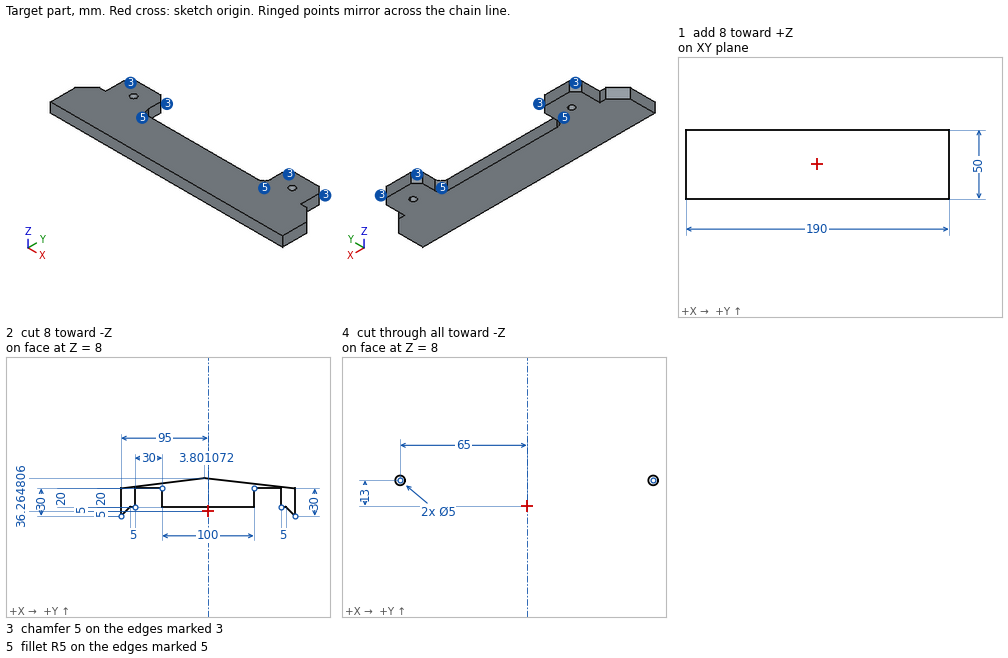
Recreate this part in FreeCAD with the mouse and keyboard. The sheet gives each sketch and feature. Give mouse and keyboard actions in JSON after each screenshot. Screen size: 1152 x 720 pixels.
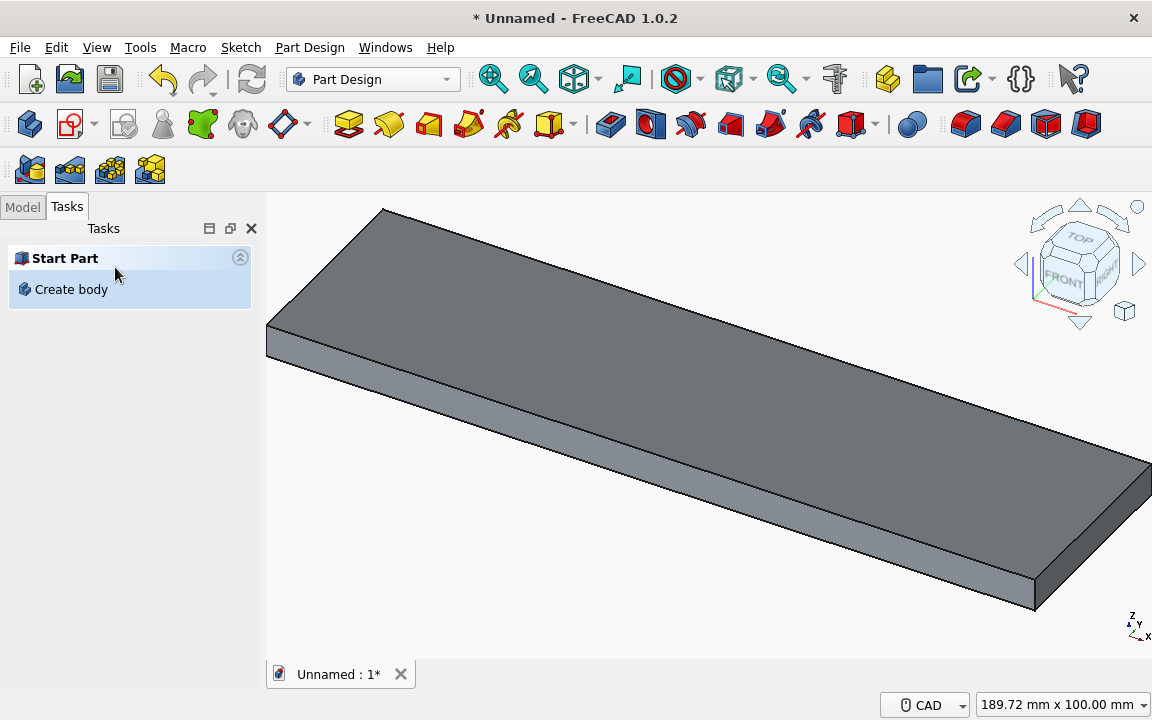
{"action": "left_click", "coordinate": [929, 466]}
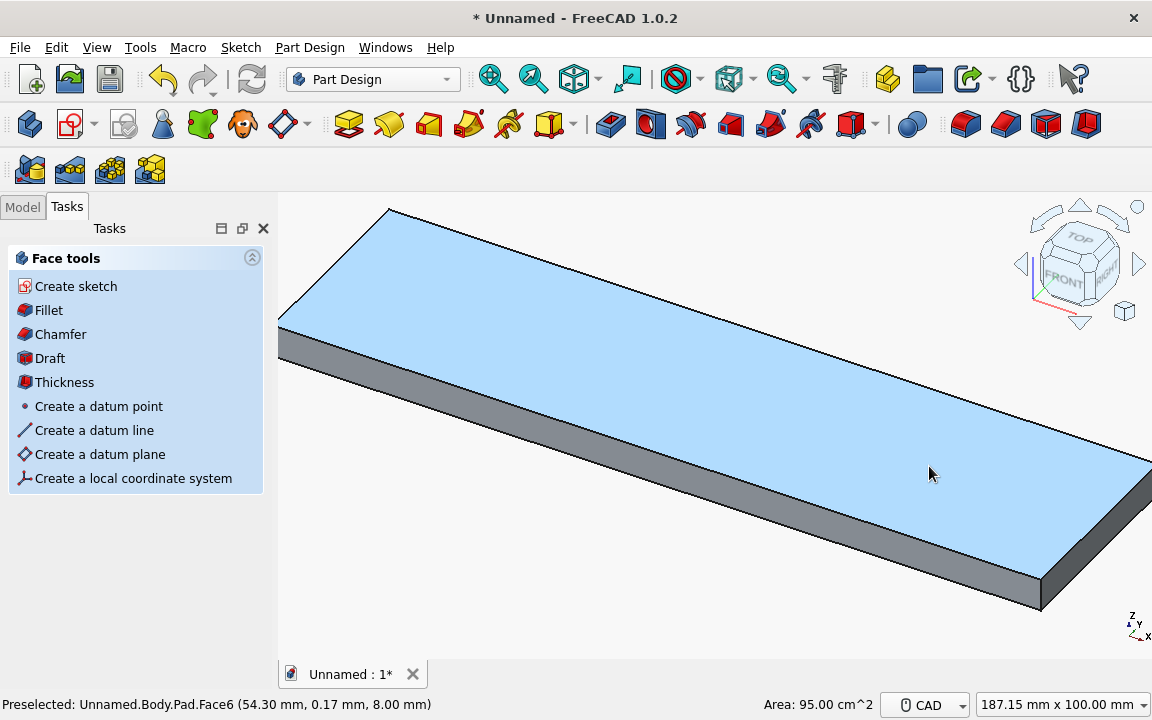
{"action": "left_click", "coordinate": [70, 124]}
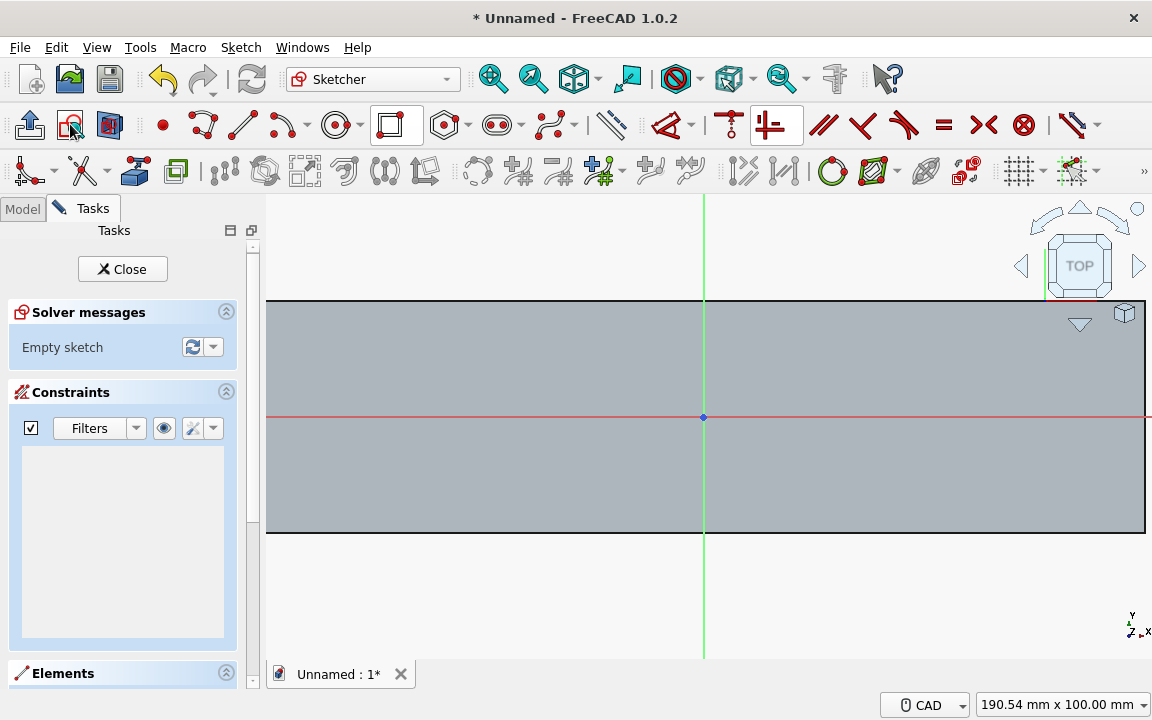
{"action": "scroll", "coordinate": [564, 526], "scroll_direction": "down", "scroll_amount": 3}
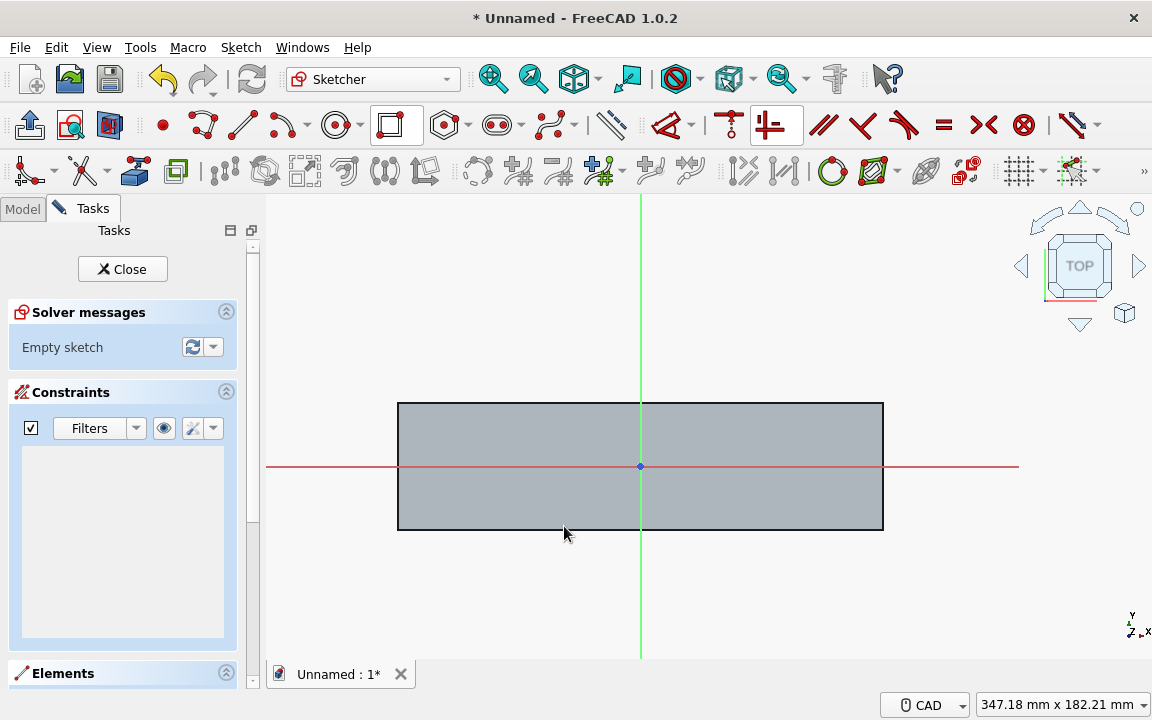
{"action": "left_click", "coordinate": [204, 126]}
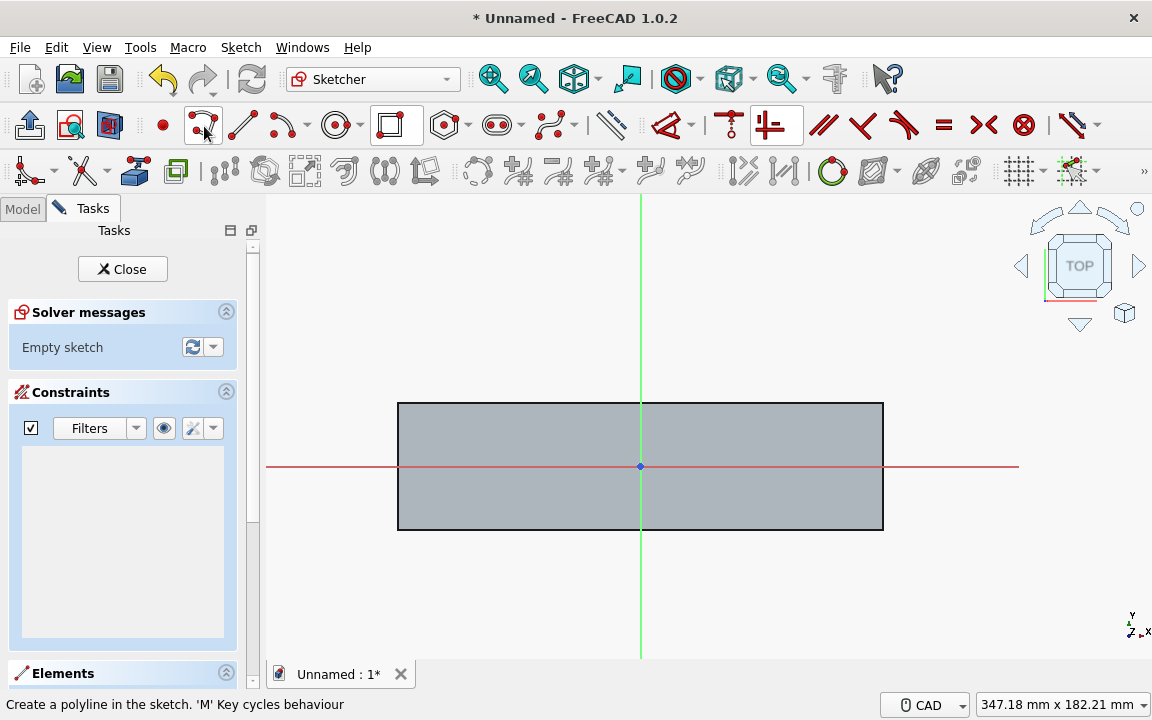
{"action": "scroll", "coordinate": [631, 374], "scroll_direction": "up", "scroll_amount": 3}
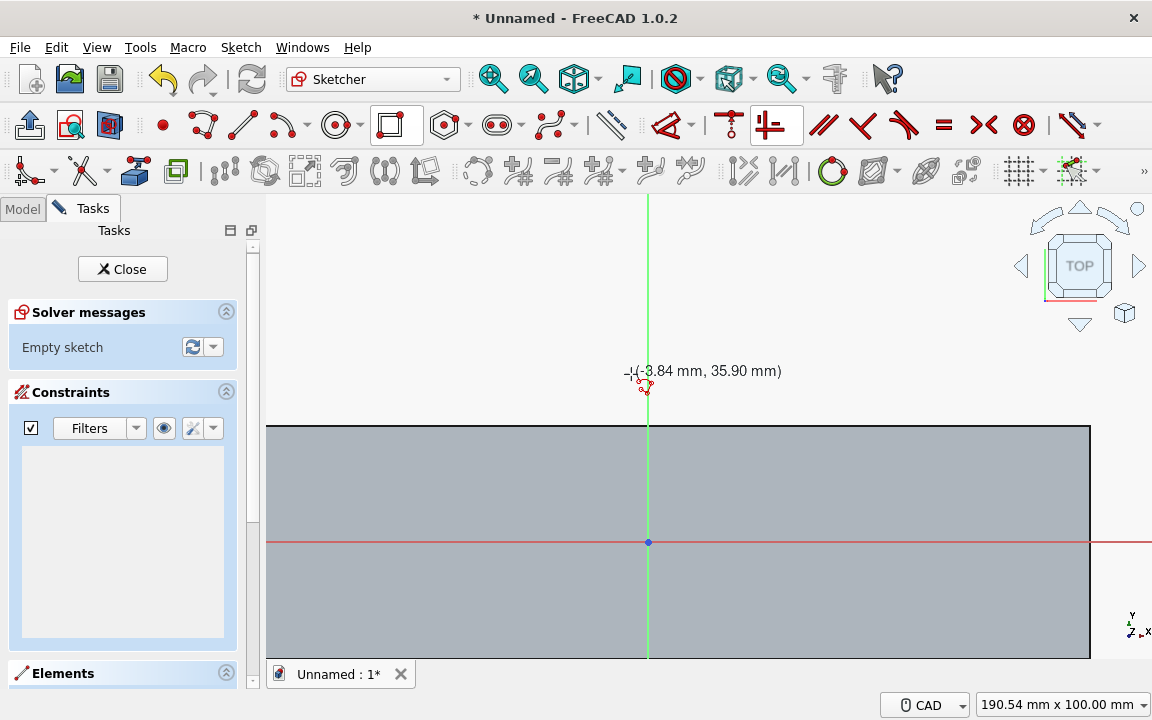
{"action": "left_click", "coordinate": [631, 374]}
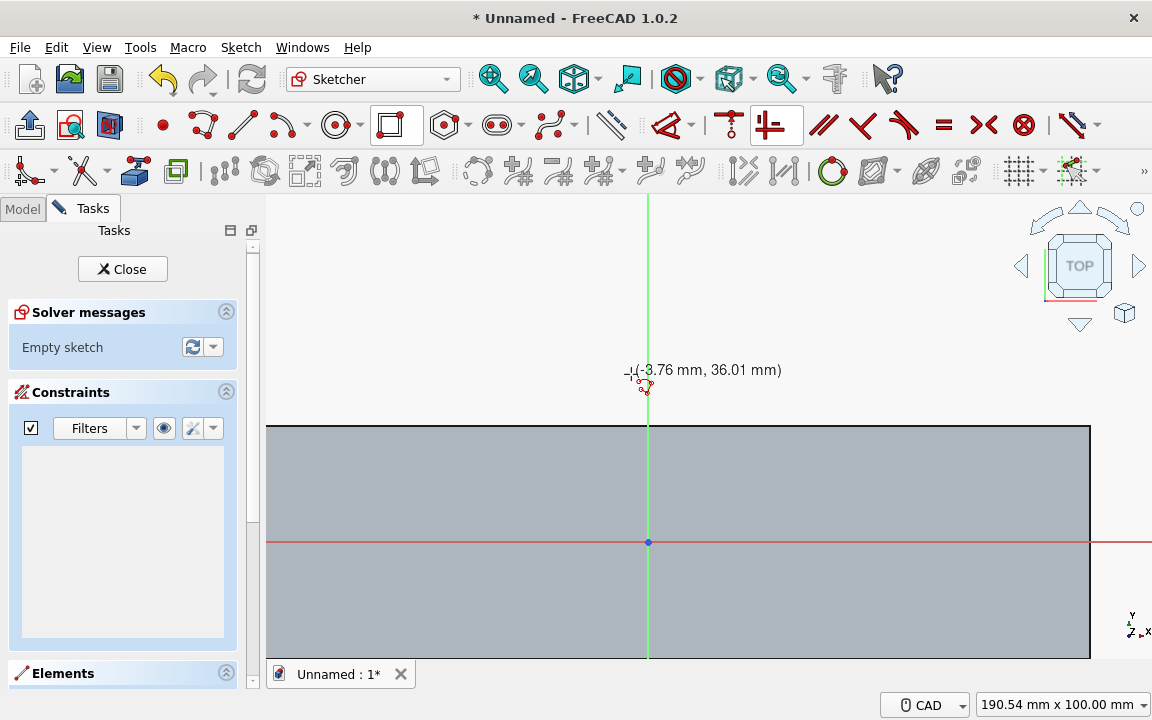
{"action": "scroll", "coordinate": [631, 374], "scroll_direction": "down", "scroll_amount": 3}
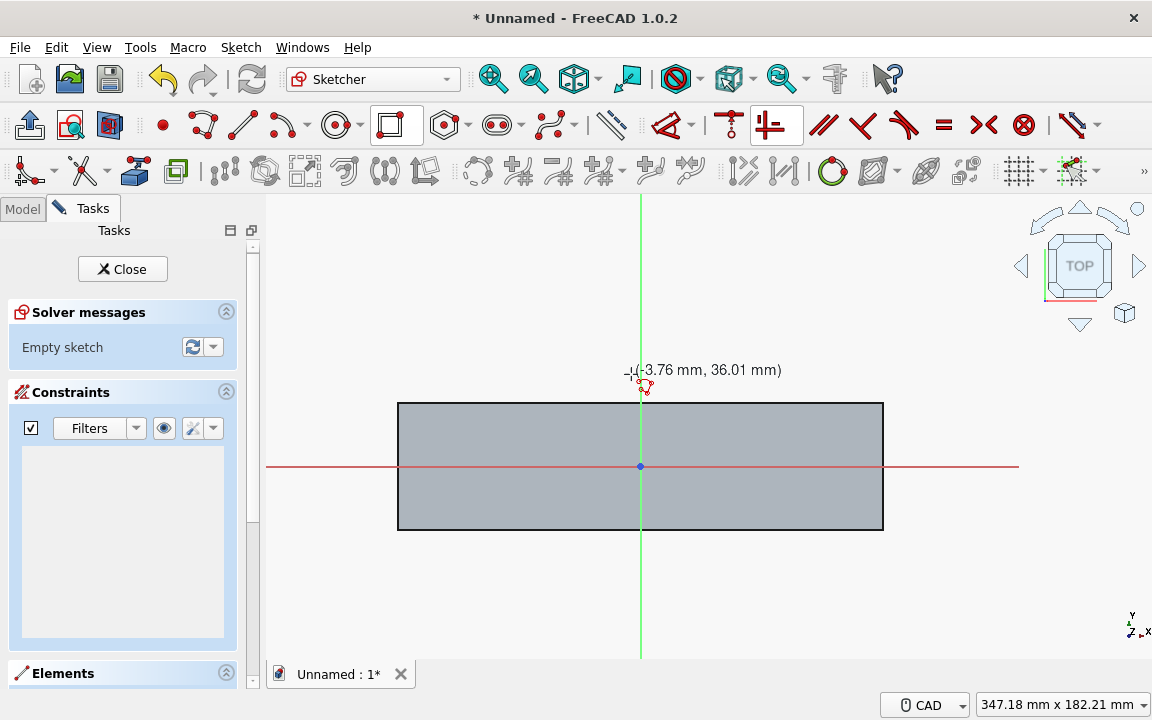
{"action": "left_click", "coordinate": [398, 403]}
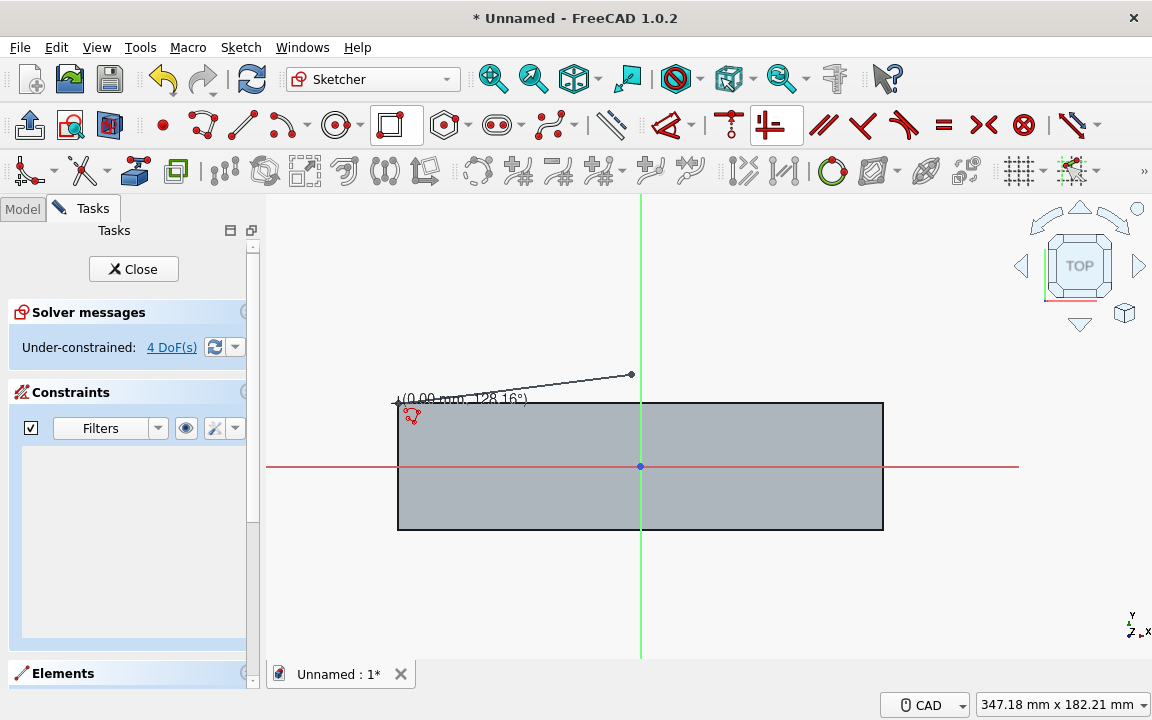
{"action": "scroll", "coordinate": [398, 479], "scroll_direction": "up", "scroll_amount": 2}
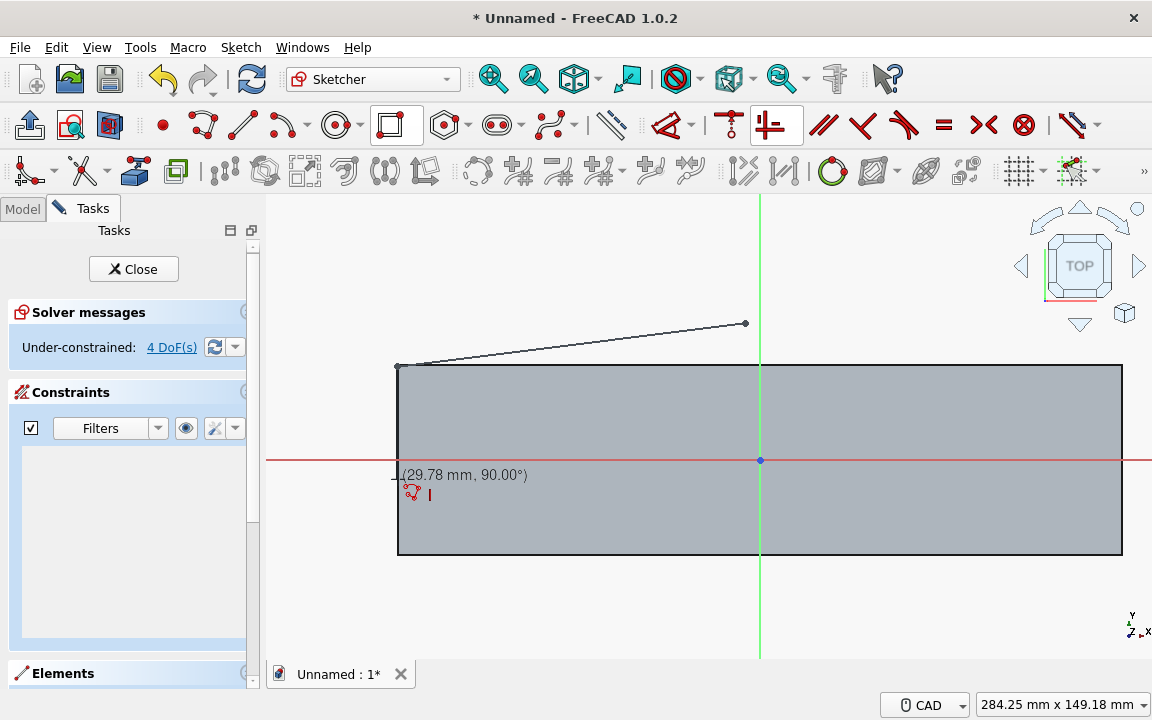
{"action": "left_click", "coordinate": [398, 479]}
{"action": "left_click", "coordinate": [437, 441]}
{"action": "left_click", "coordinate": [456, 441]}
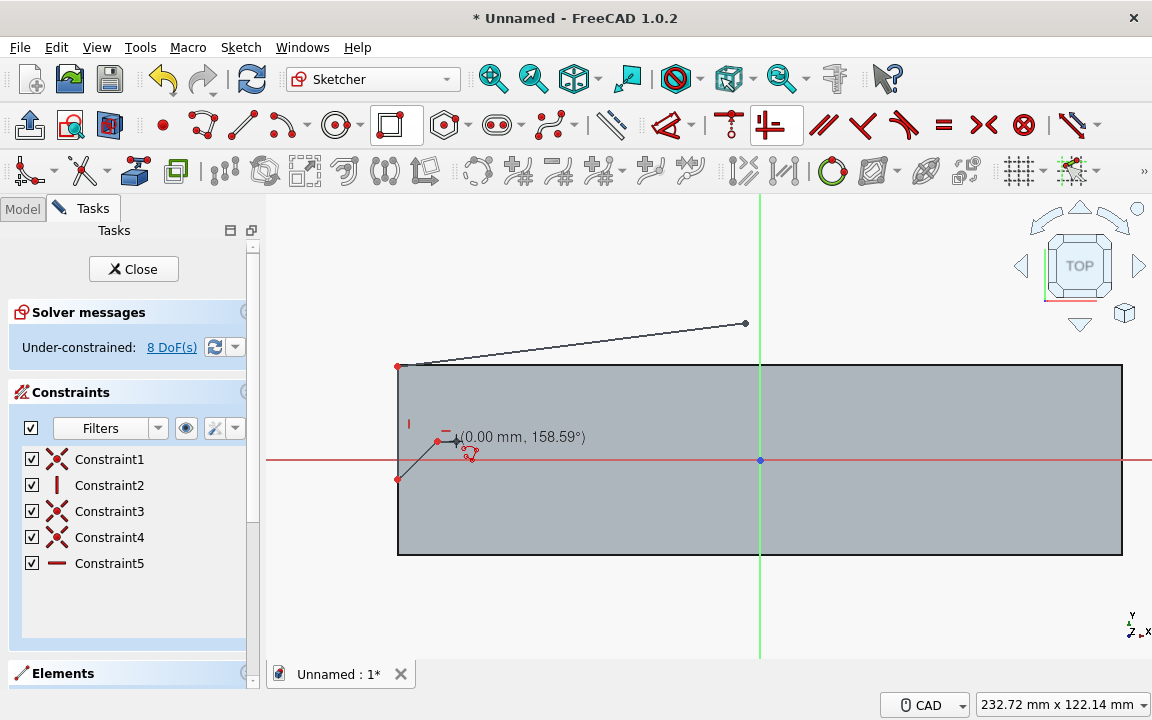
{"action": "scroll", "coordinate": [456, 365], "scroll_direction": "up", "scroll_amount": 5}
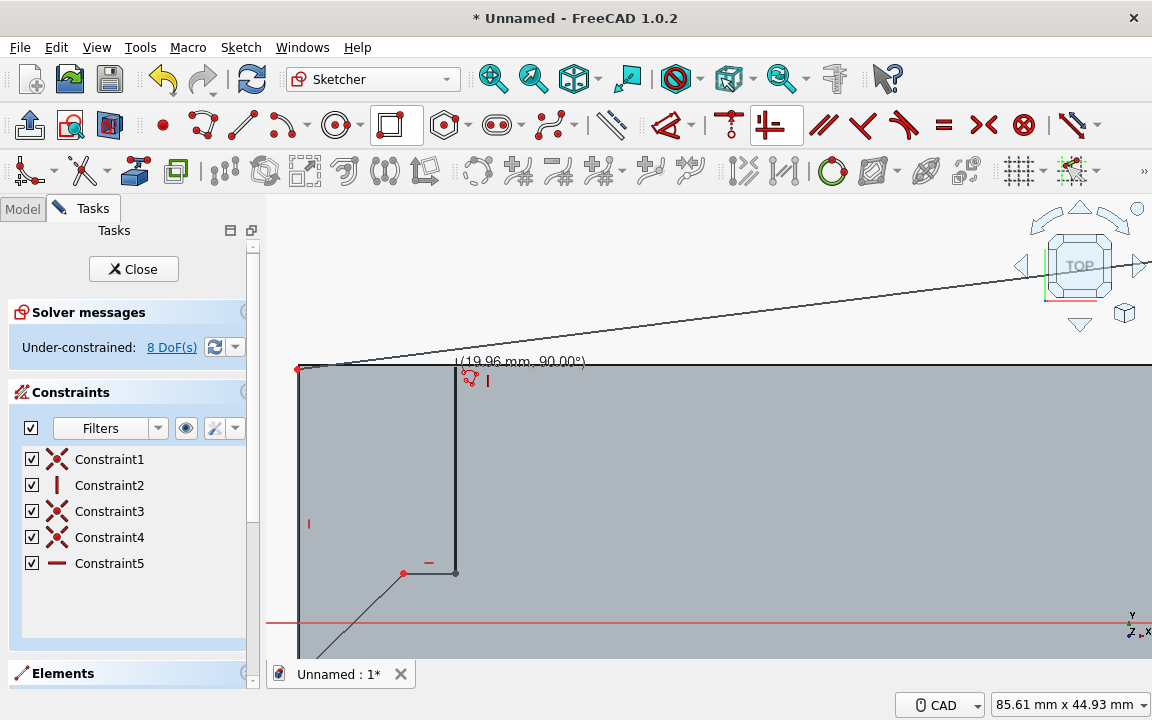
{"action": "left_click", "coordinate": [456, 365]}